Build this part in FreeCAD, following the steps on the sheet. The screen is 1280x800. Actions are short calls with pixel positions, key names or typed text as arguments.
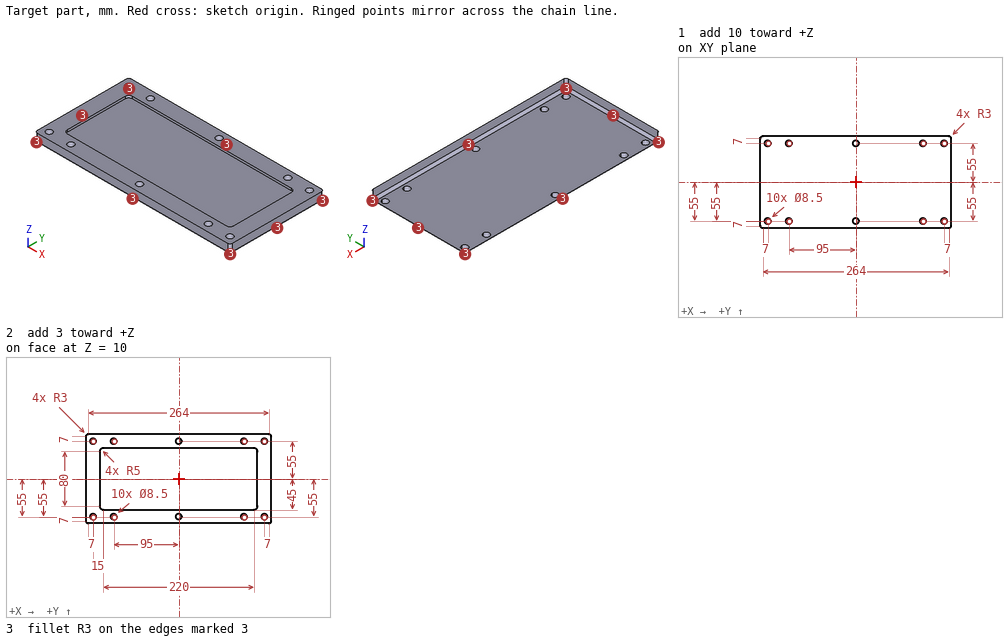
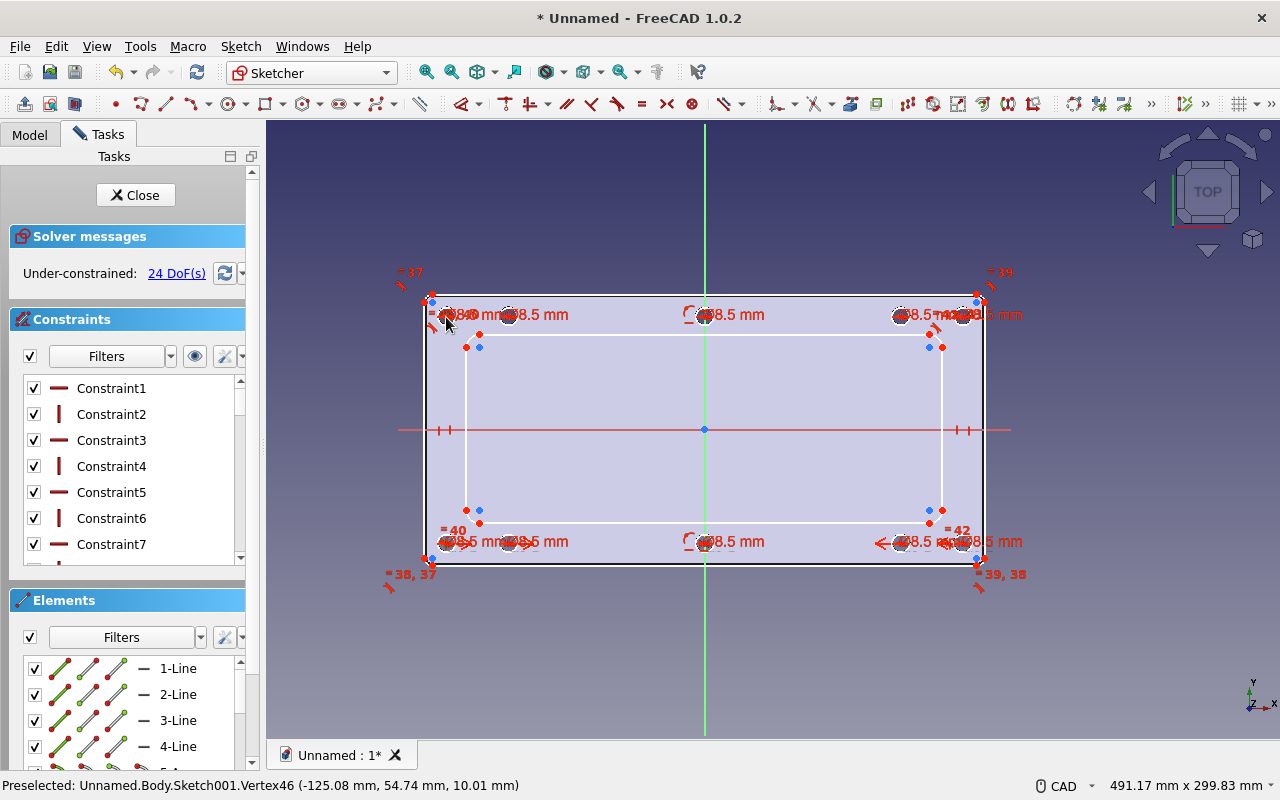
click(529, 430)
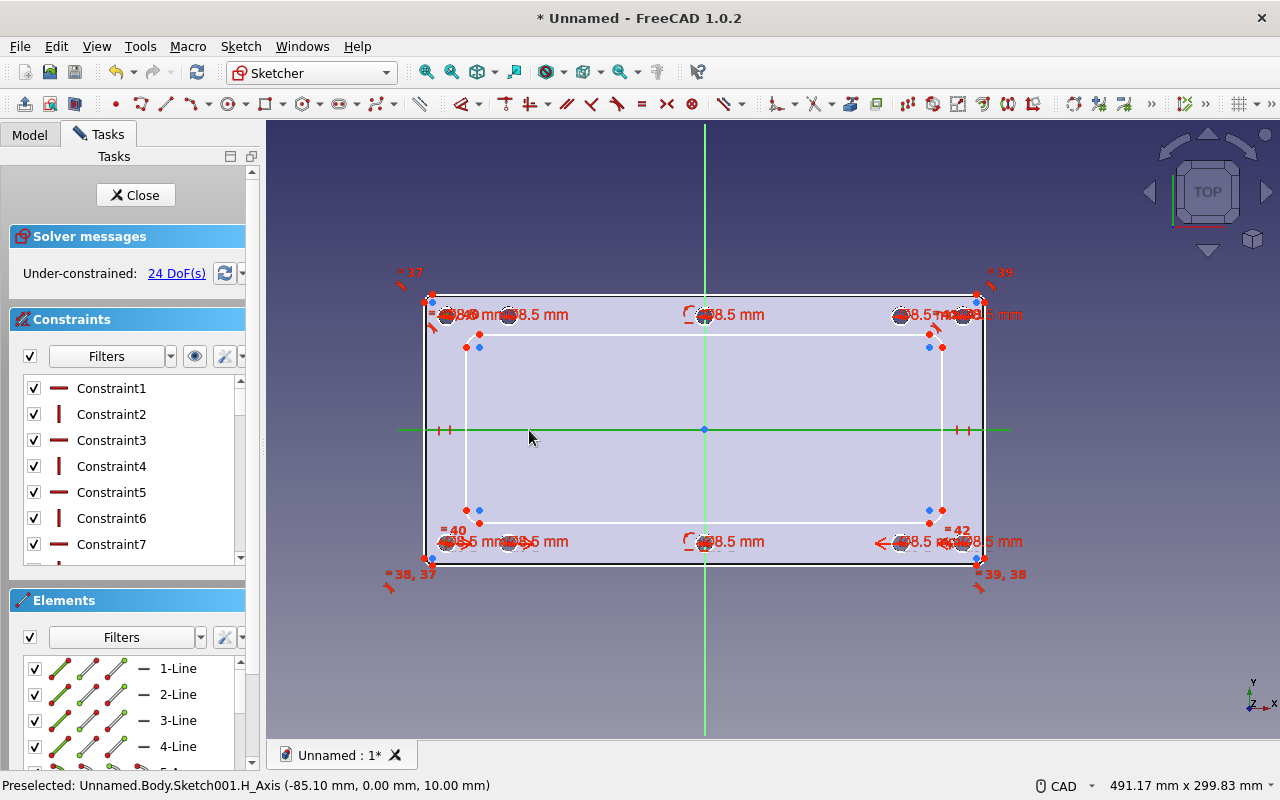
click(667, 104)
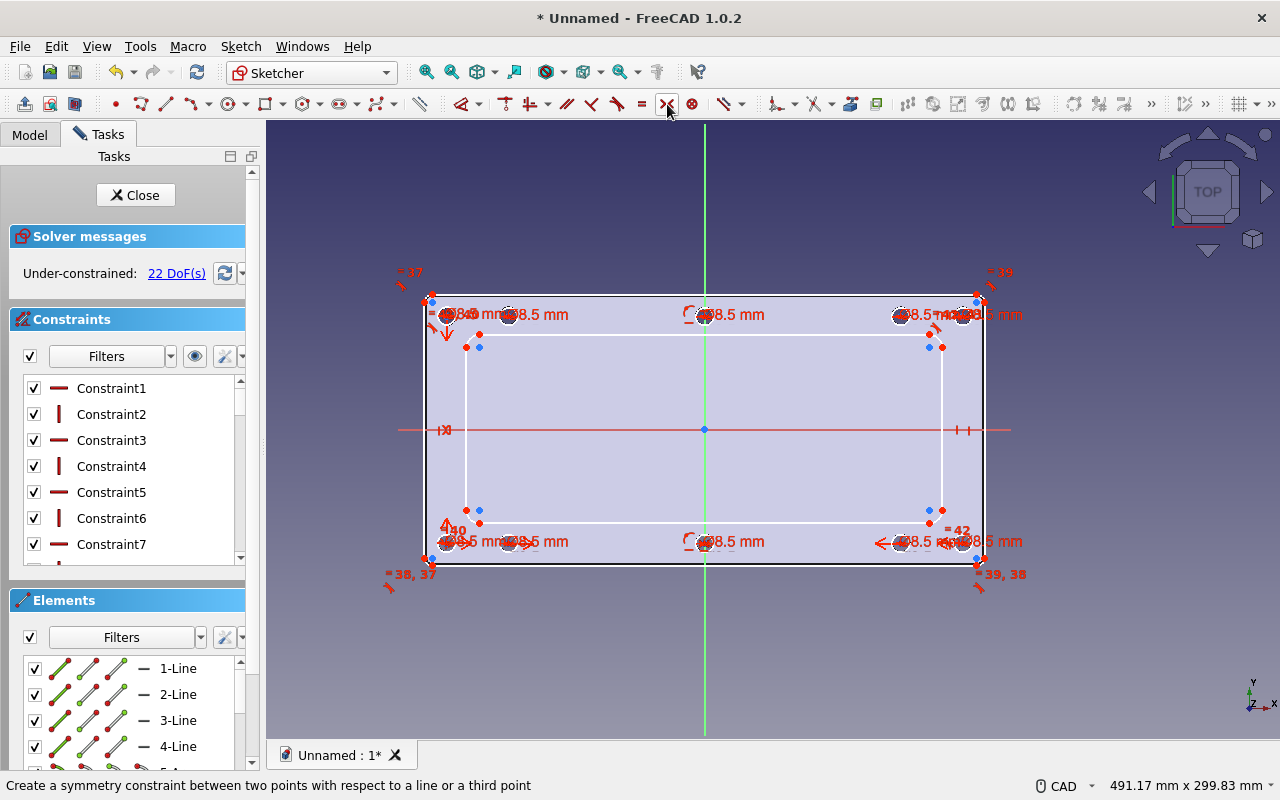
click(509, 544)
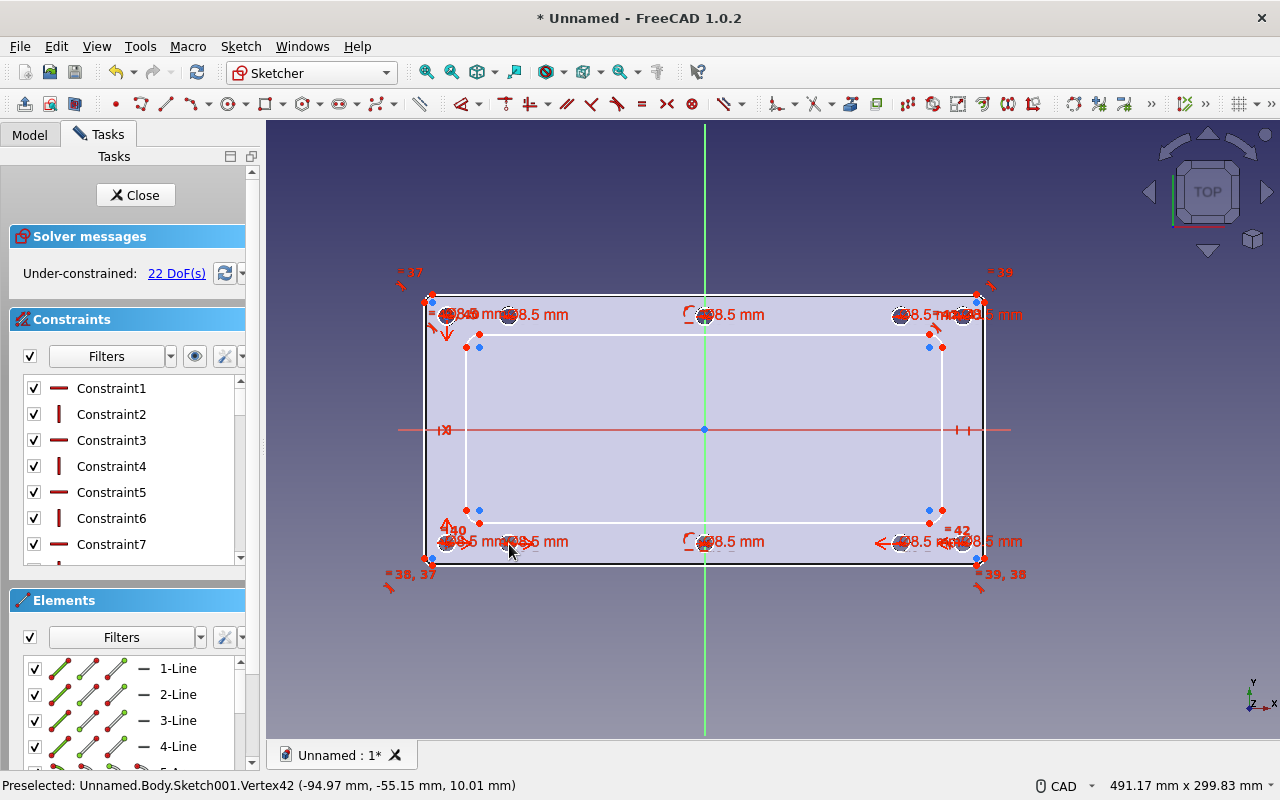
click(509, 317)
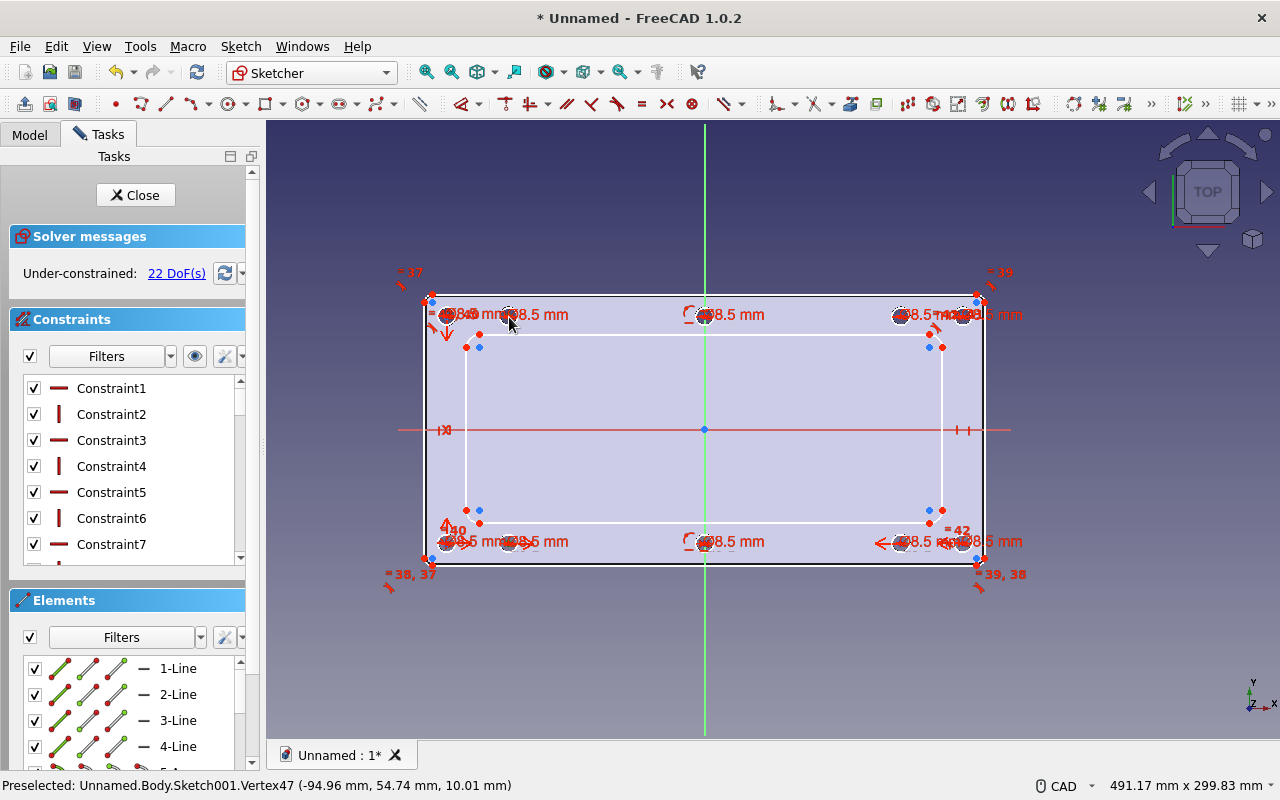
click(529, 430)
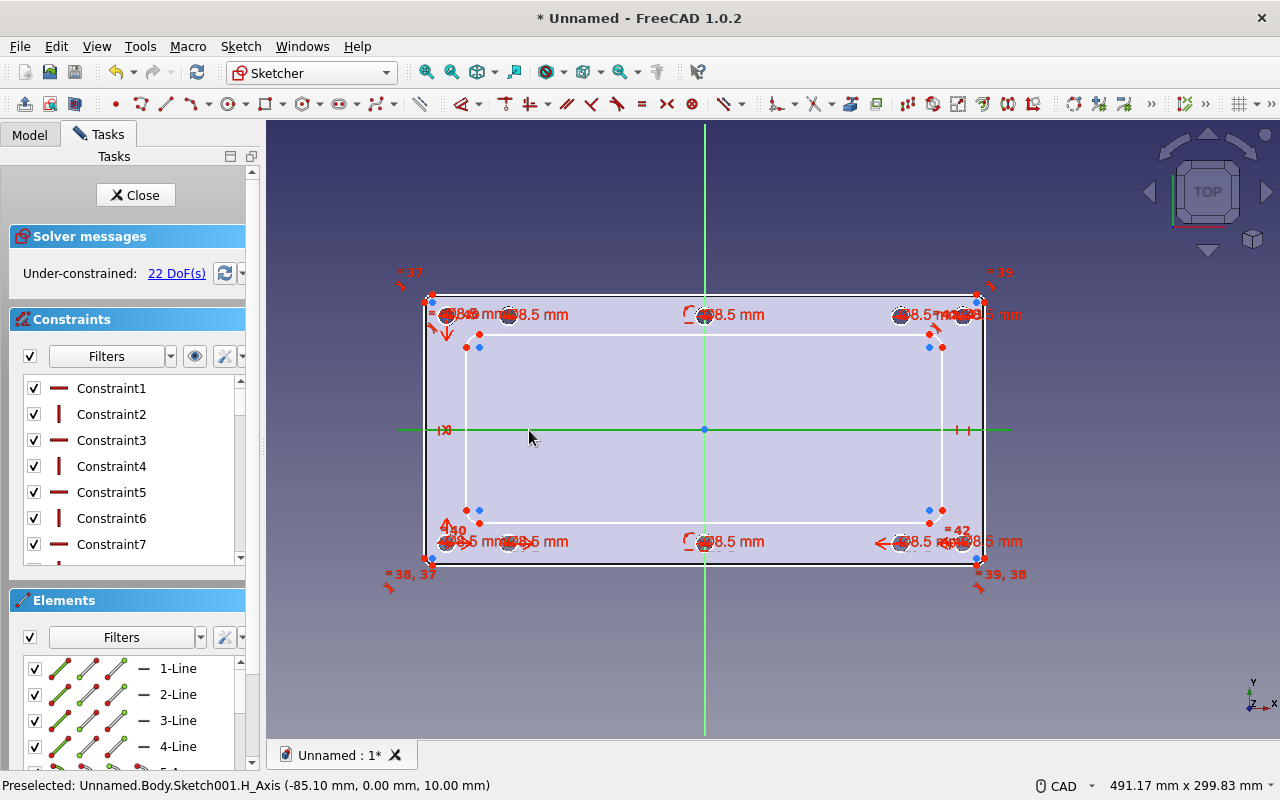
click(667, 104)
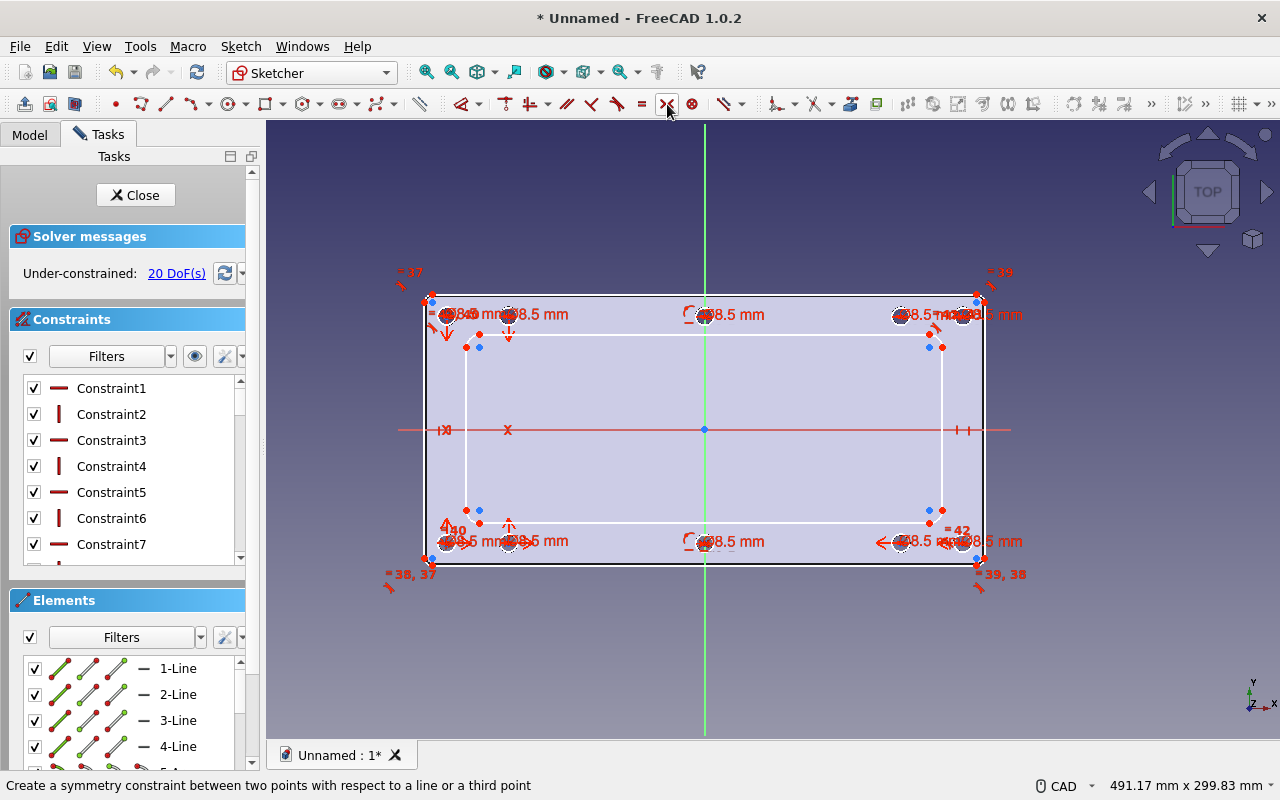
click(901, 543)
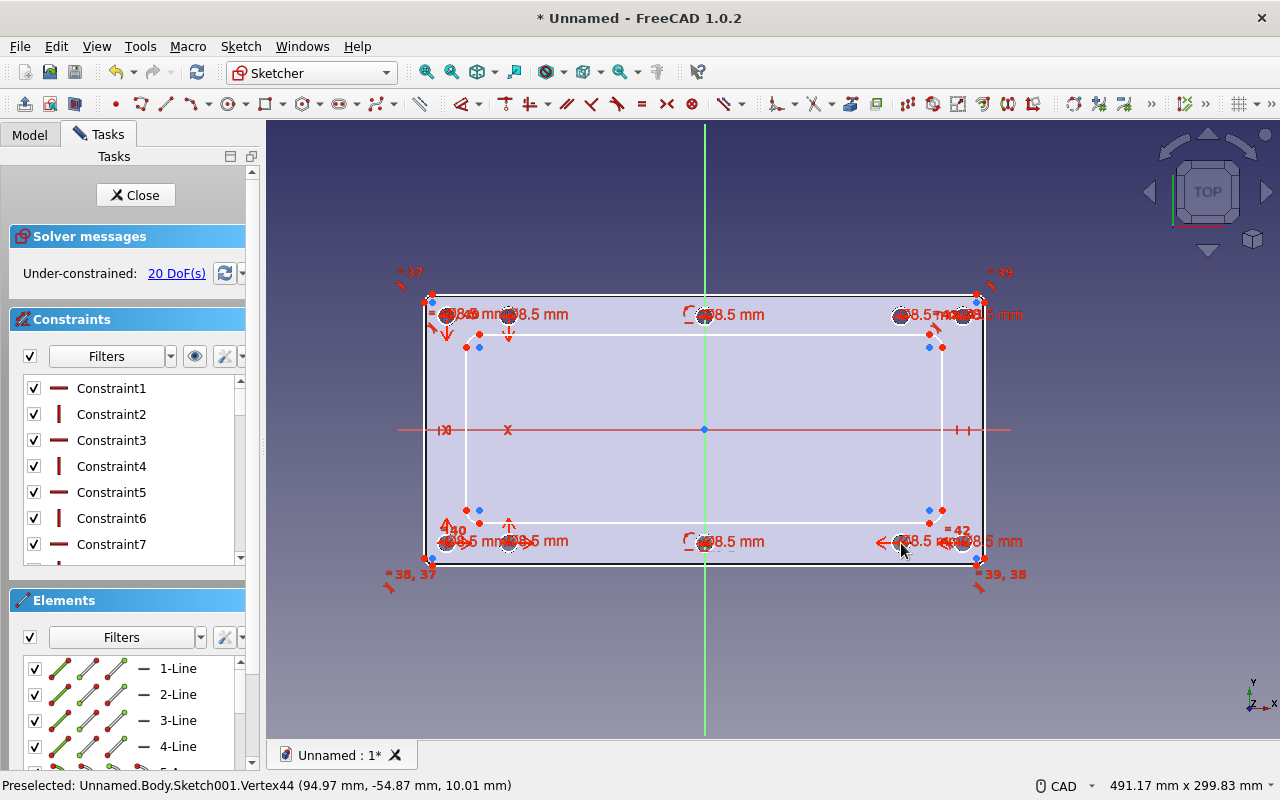
click(901, 317)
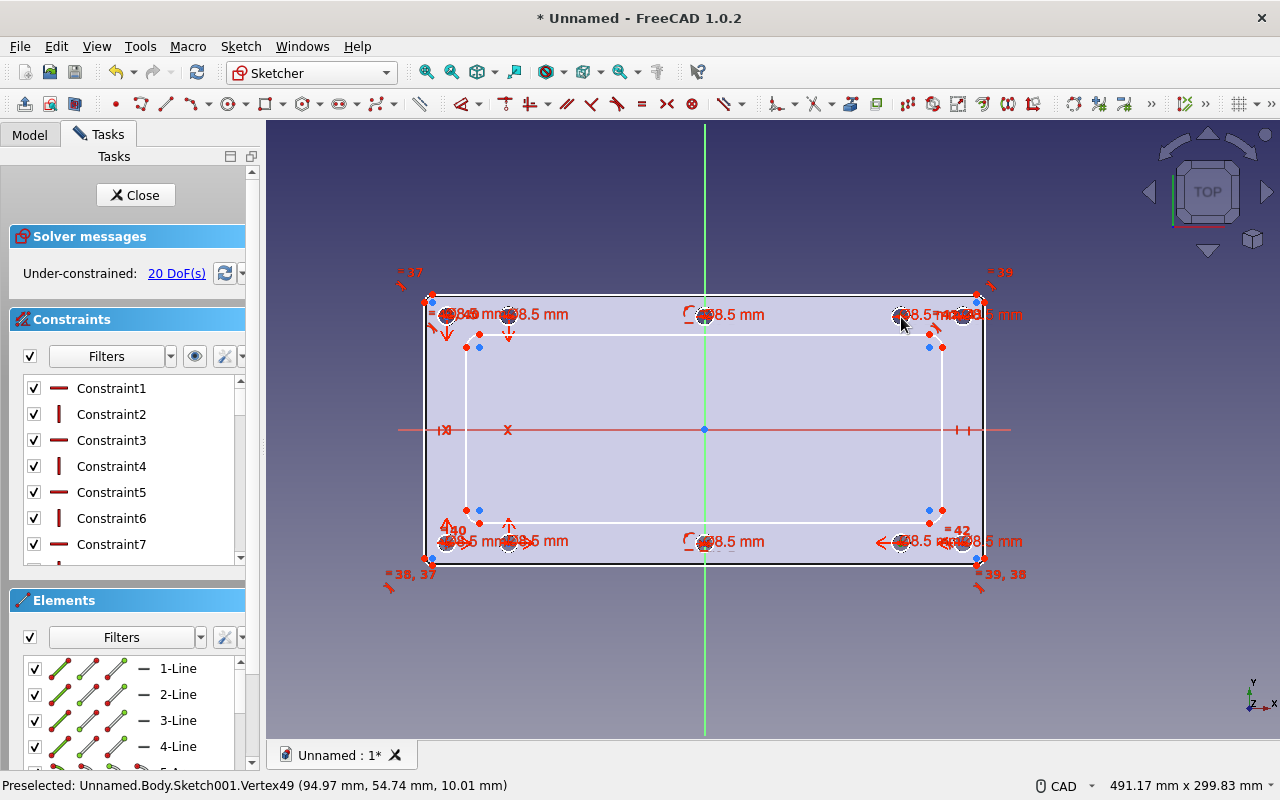
click(529, 430)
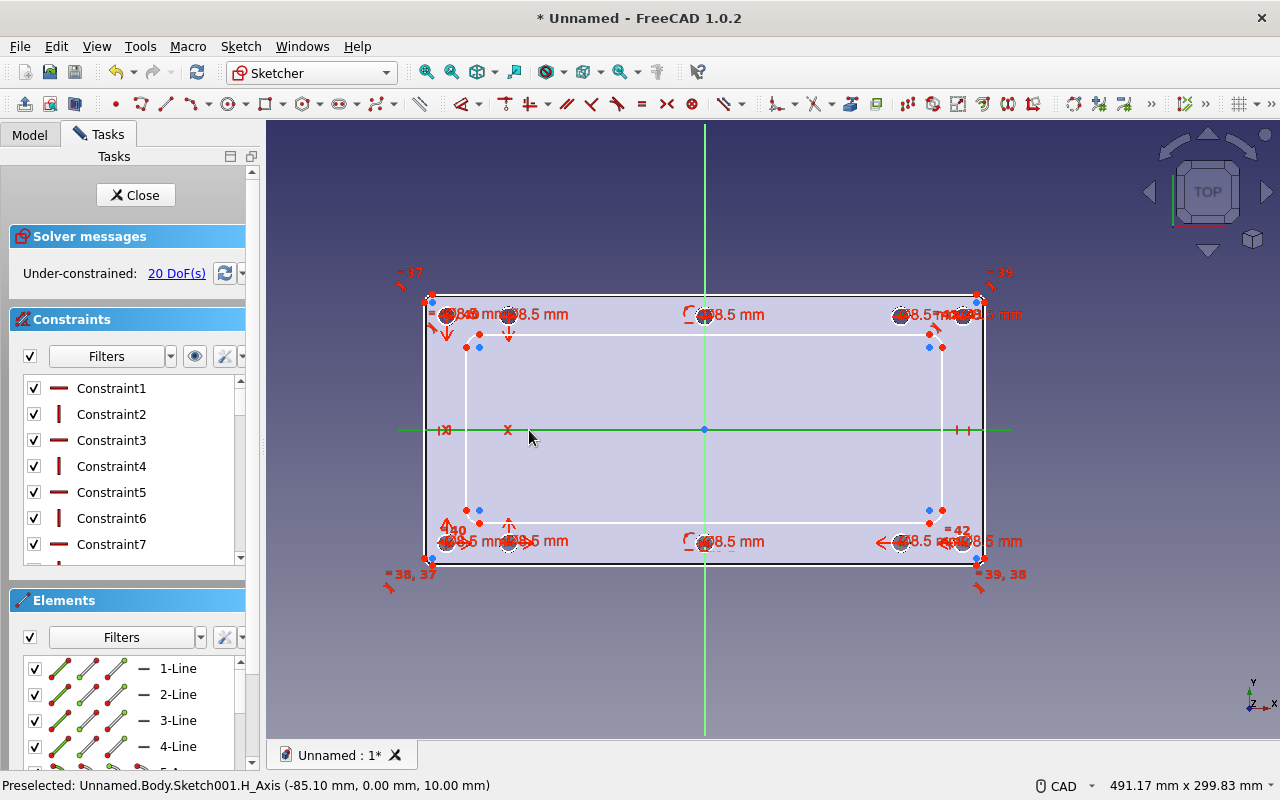
click(667, 104)